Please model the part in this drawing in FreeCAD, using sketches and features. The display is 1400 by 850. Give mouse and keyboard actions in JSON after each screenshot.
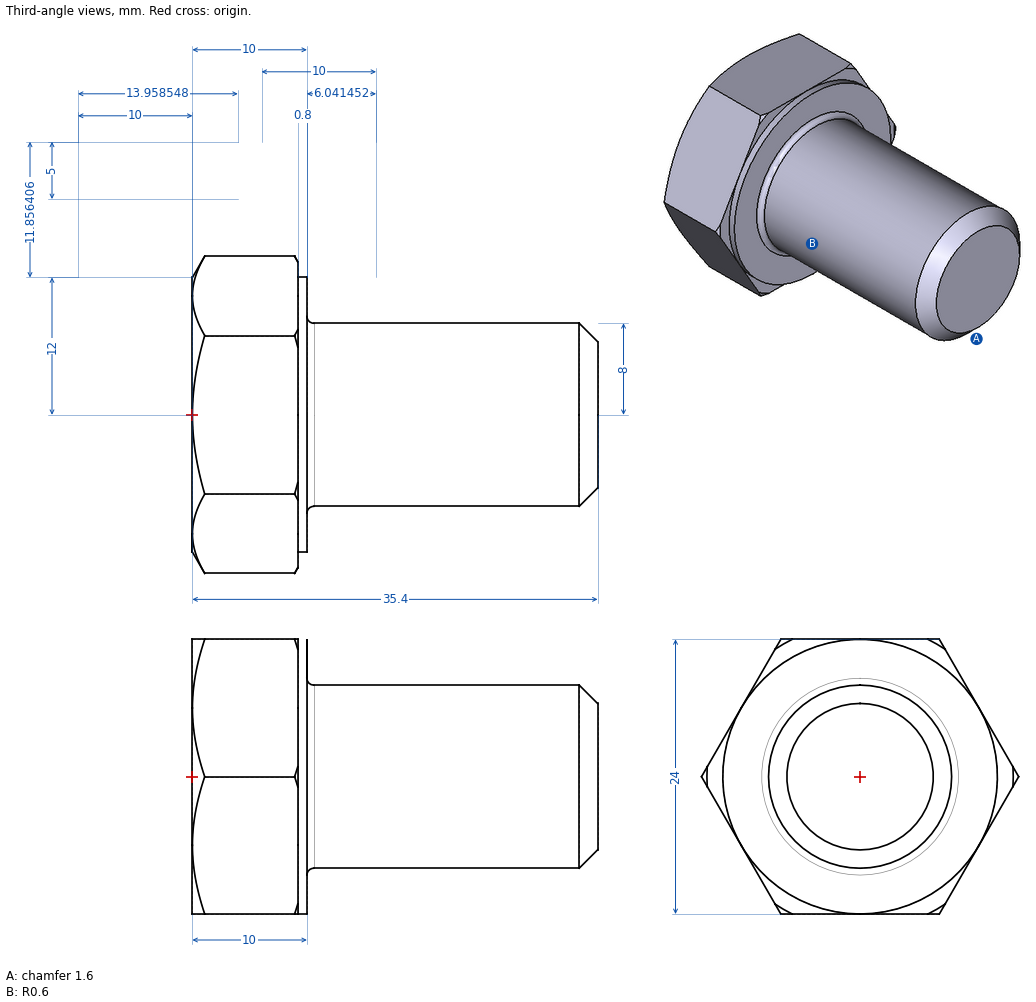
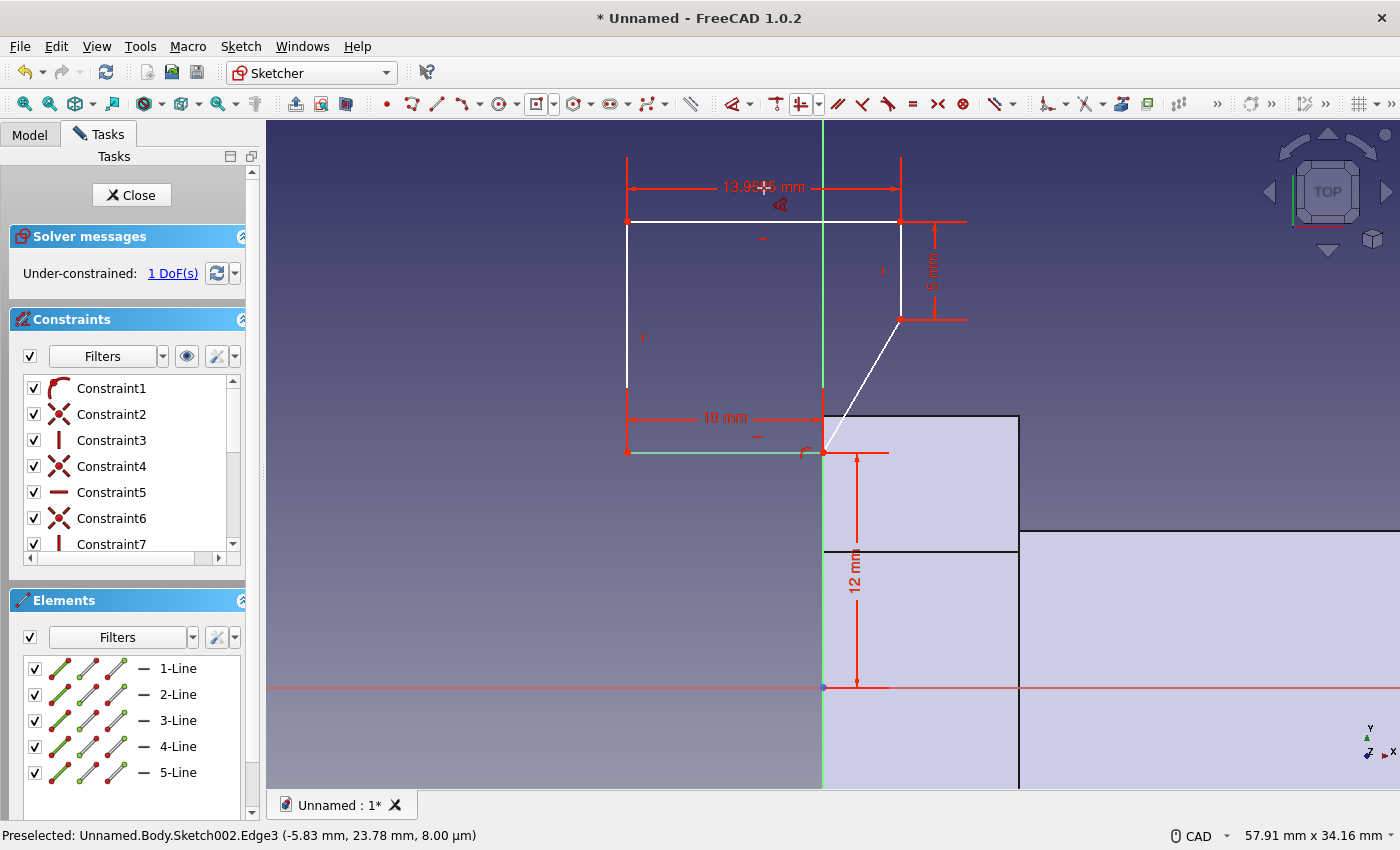
{"action": "left_click", "coordinate": [627, 291]}
{"action": "left_click", "coordinate": [593, 337]}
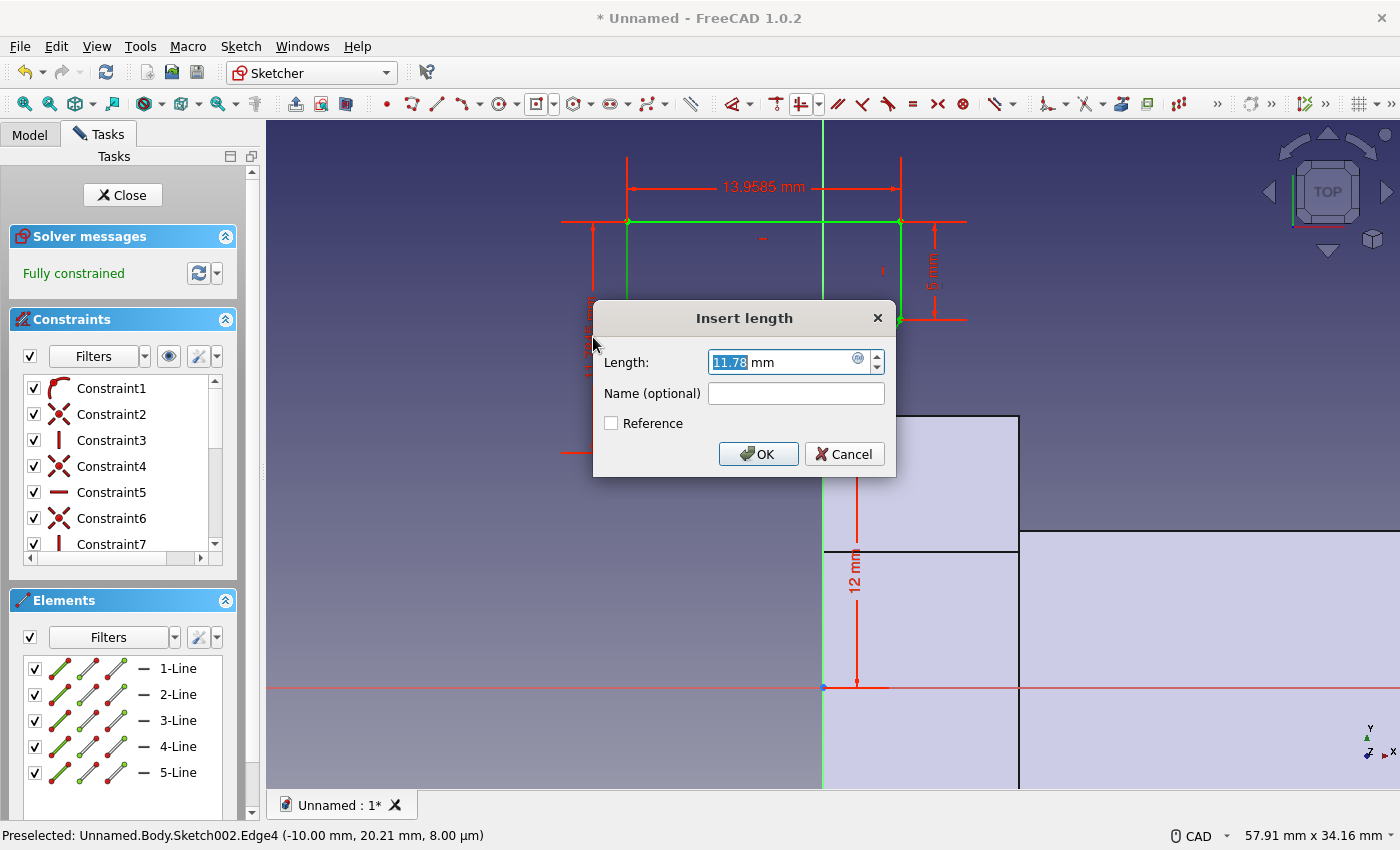
{"action": "type", "text": "11.856406"}
{"action": "key", "text": "Return"}
{"action": "key", "text": "Escape"}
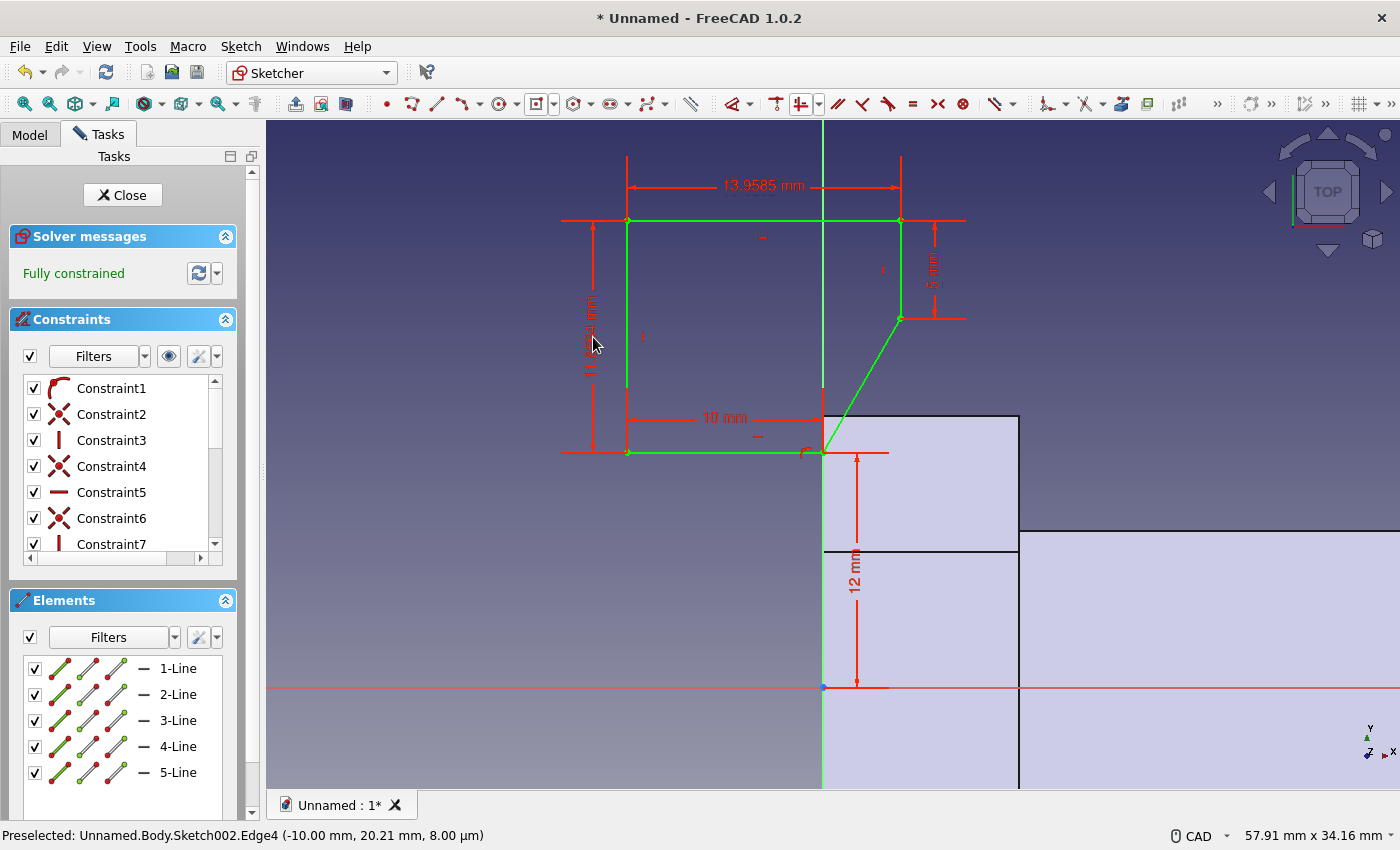
{"action": "left_click", "coordinate": [123, 195]}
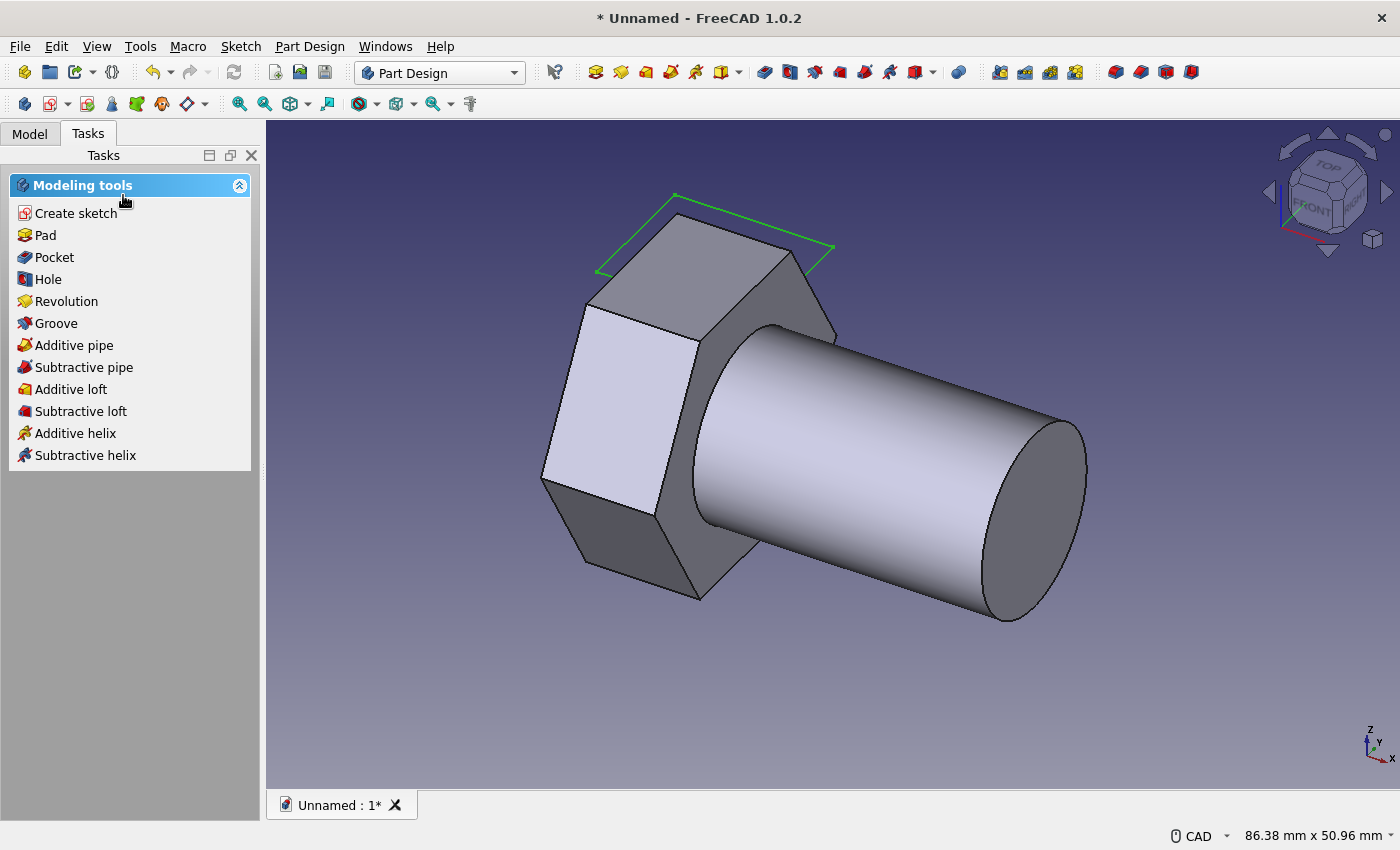
{"action": "left_click", "coordinate": [815, 72]}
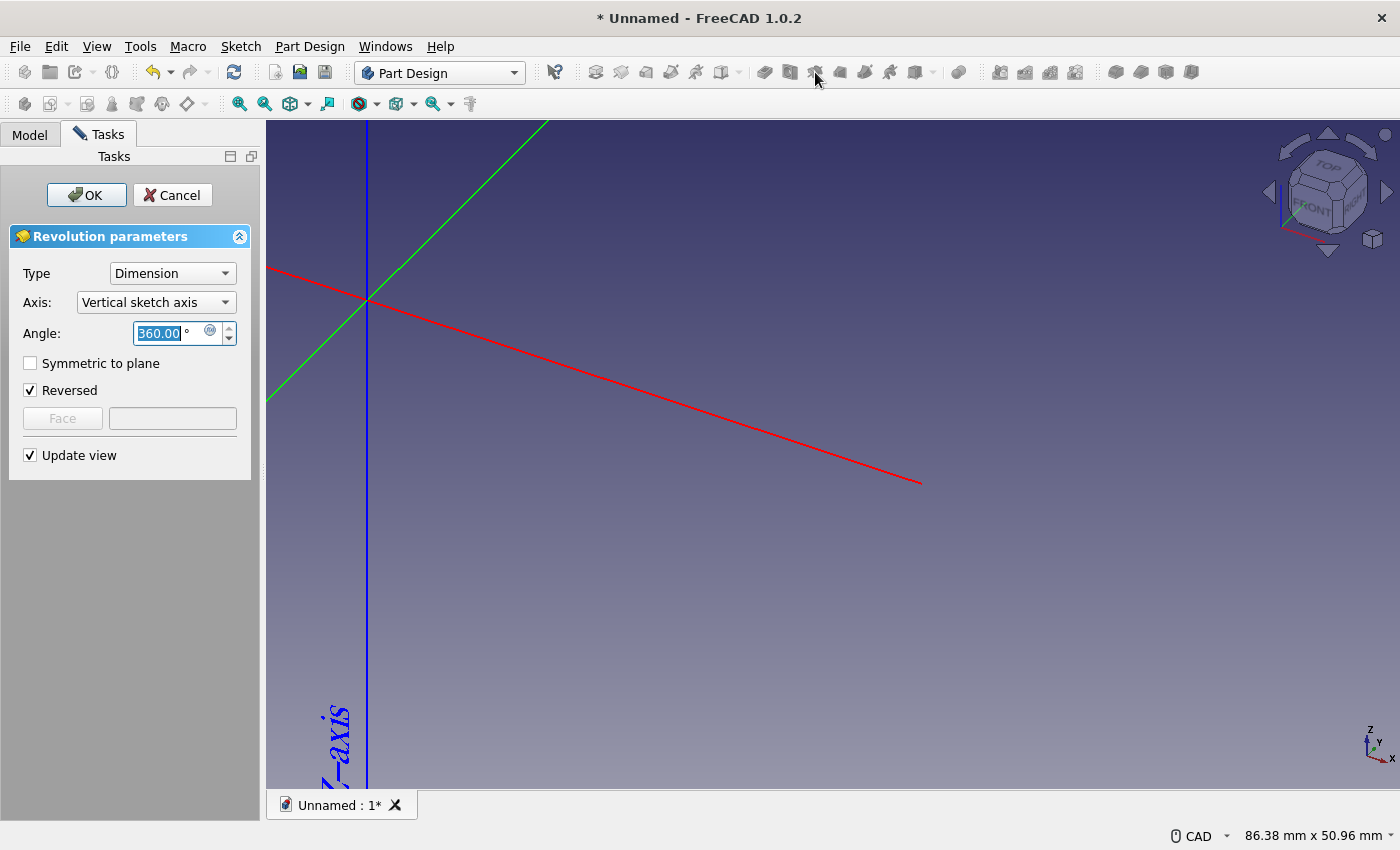
{"action": "left_click", "coordinate": [157, 302]}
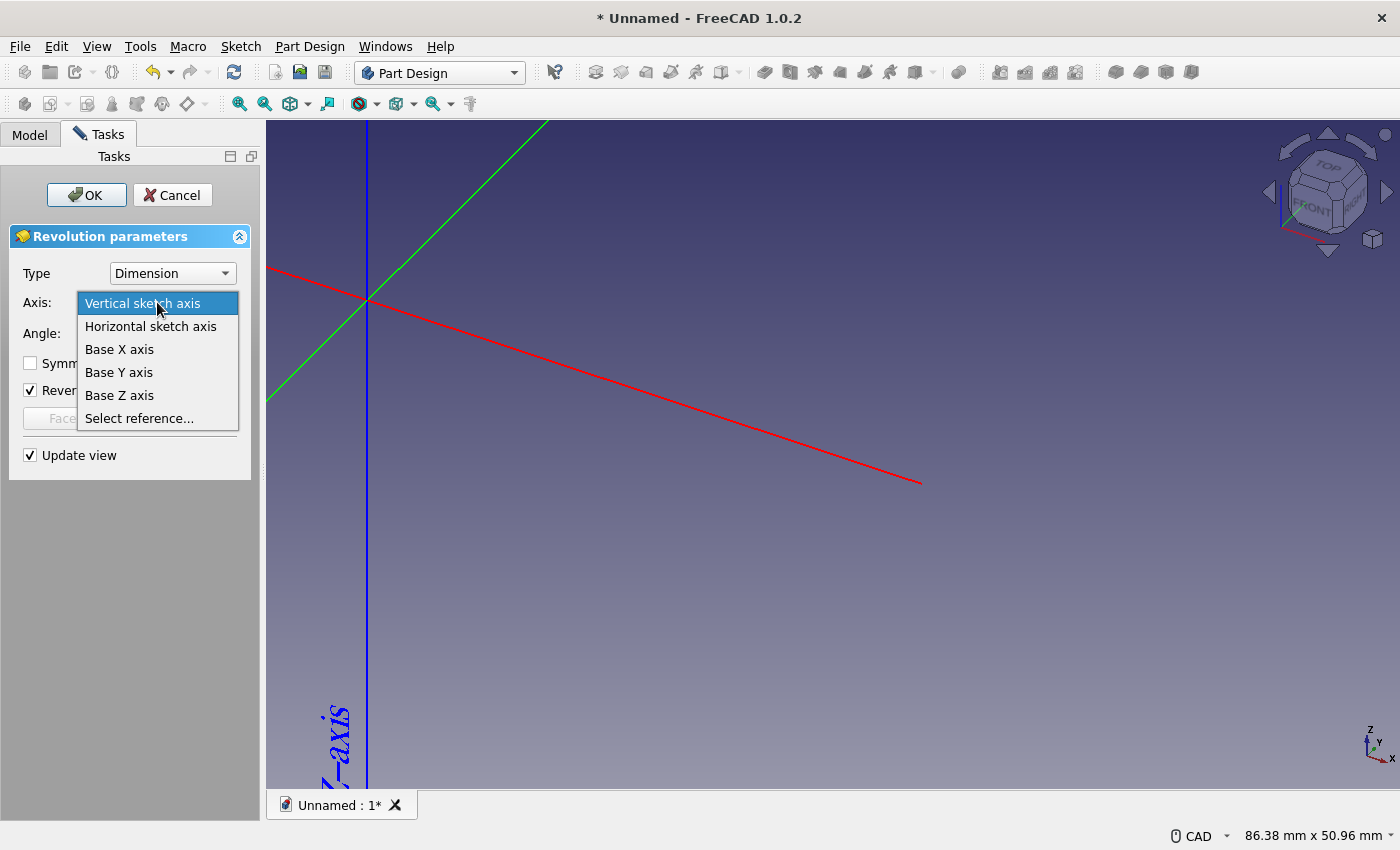
{"action": "left_click", "coordinate": [156, 326]}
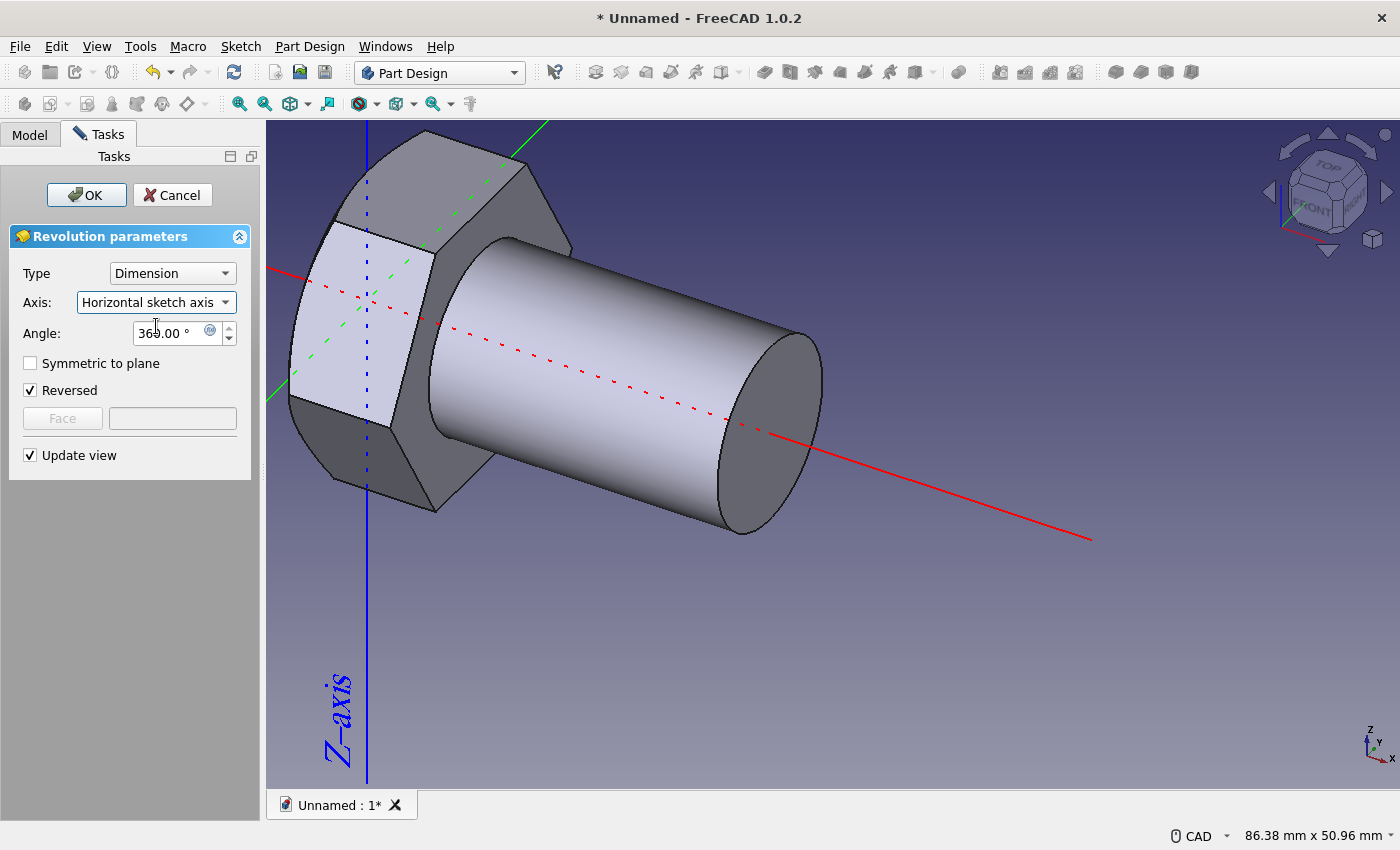
{"action": "left_click", "coordinate": [87, 195]}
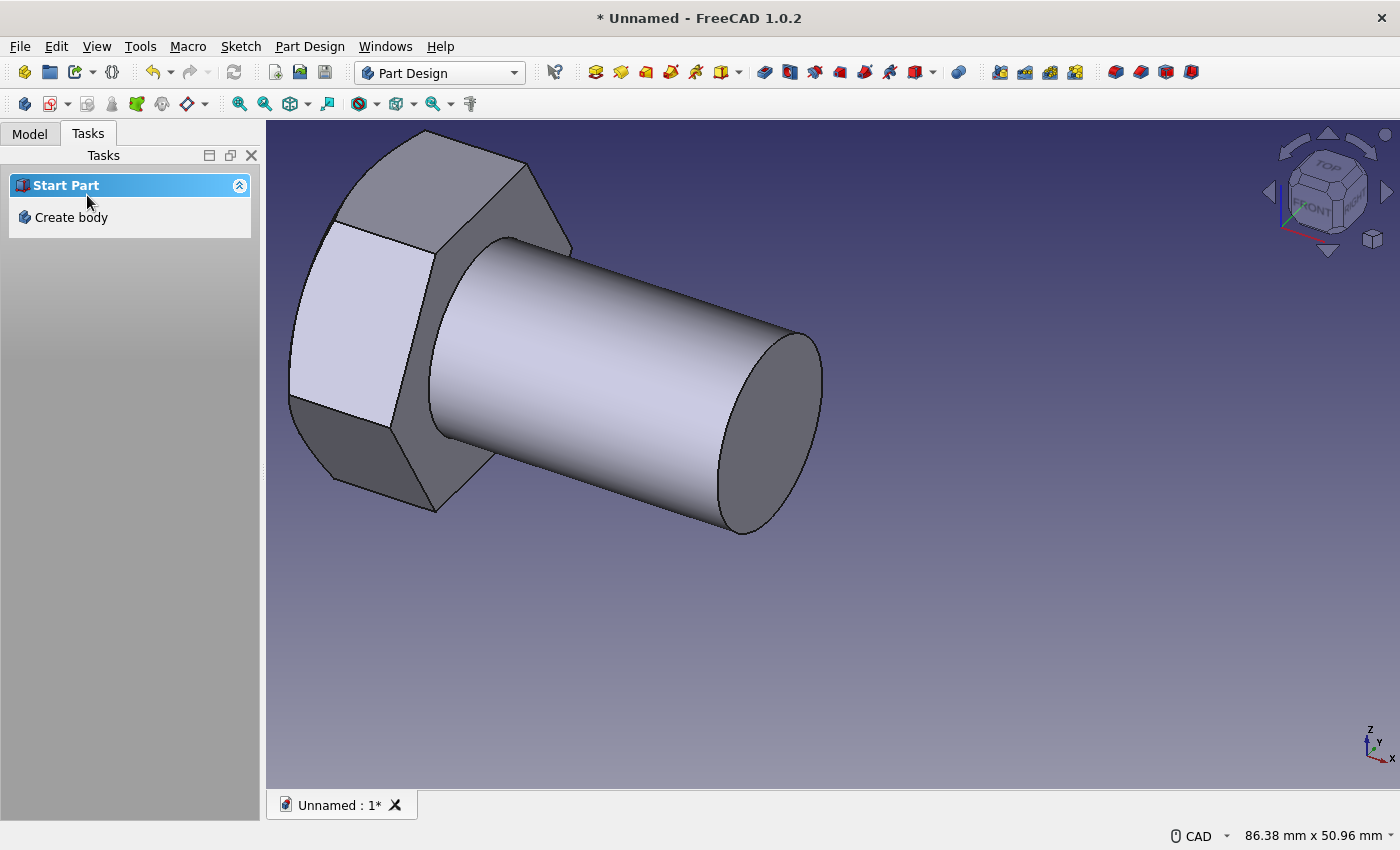
{"action": "left_click", "coordinate": [240, 104]}